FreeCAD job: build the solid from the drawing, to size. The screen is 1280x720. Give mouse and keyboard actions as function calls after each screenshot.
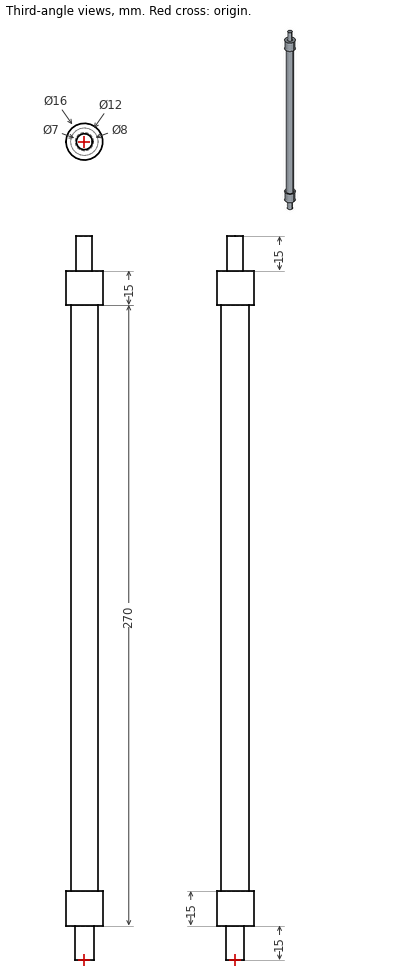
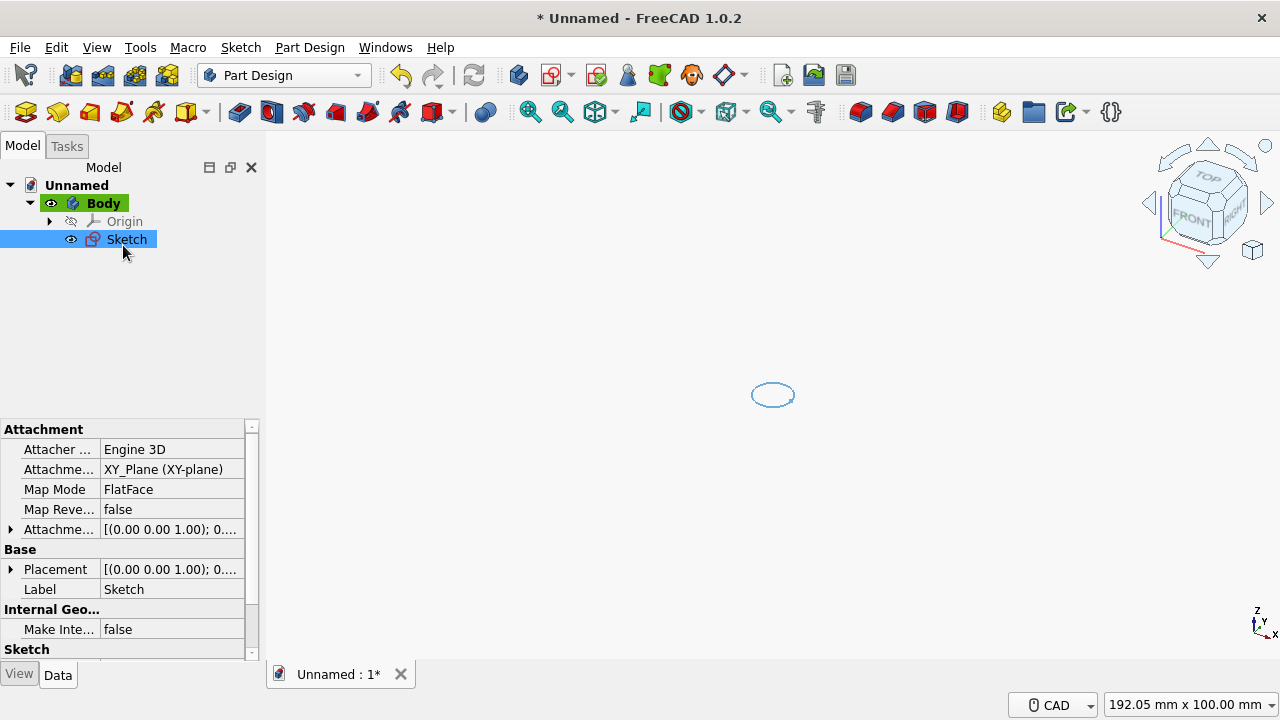
click(26, 112)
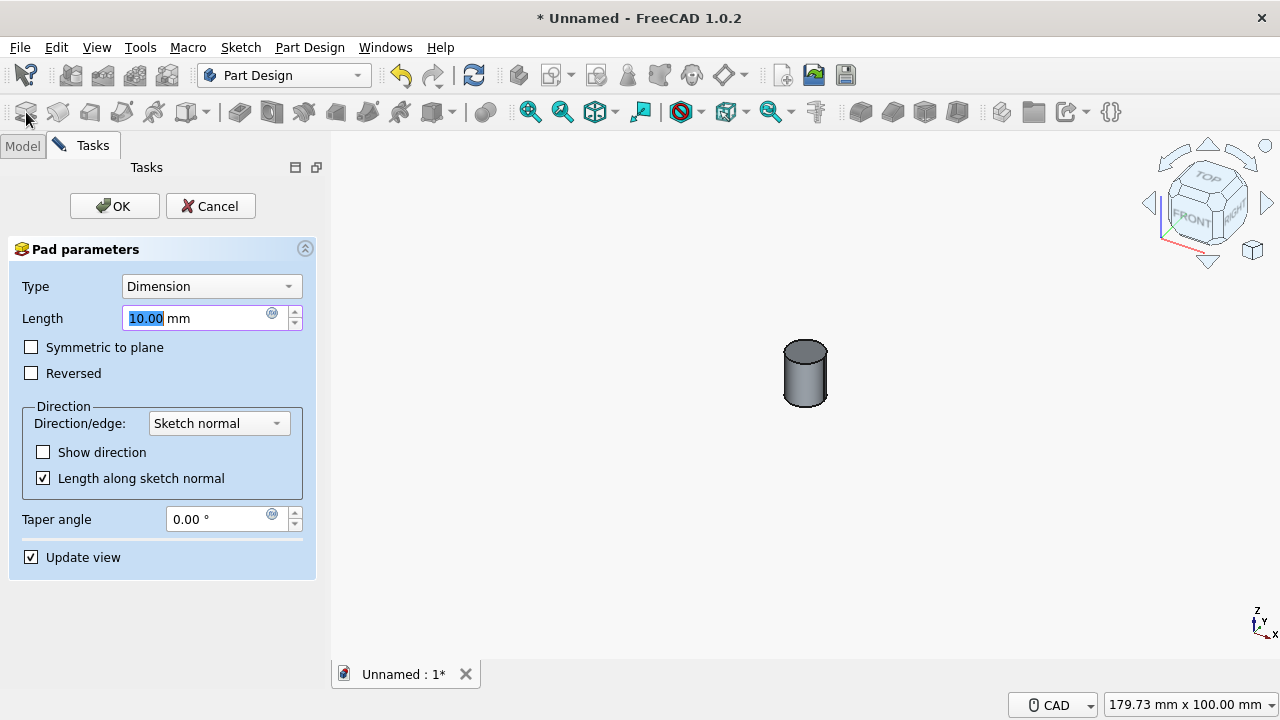
text(15)
key(Tab)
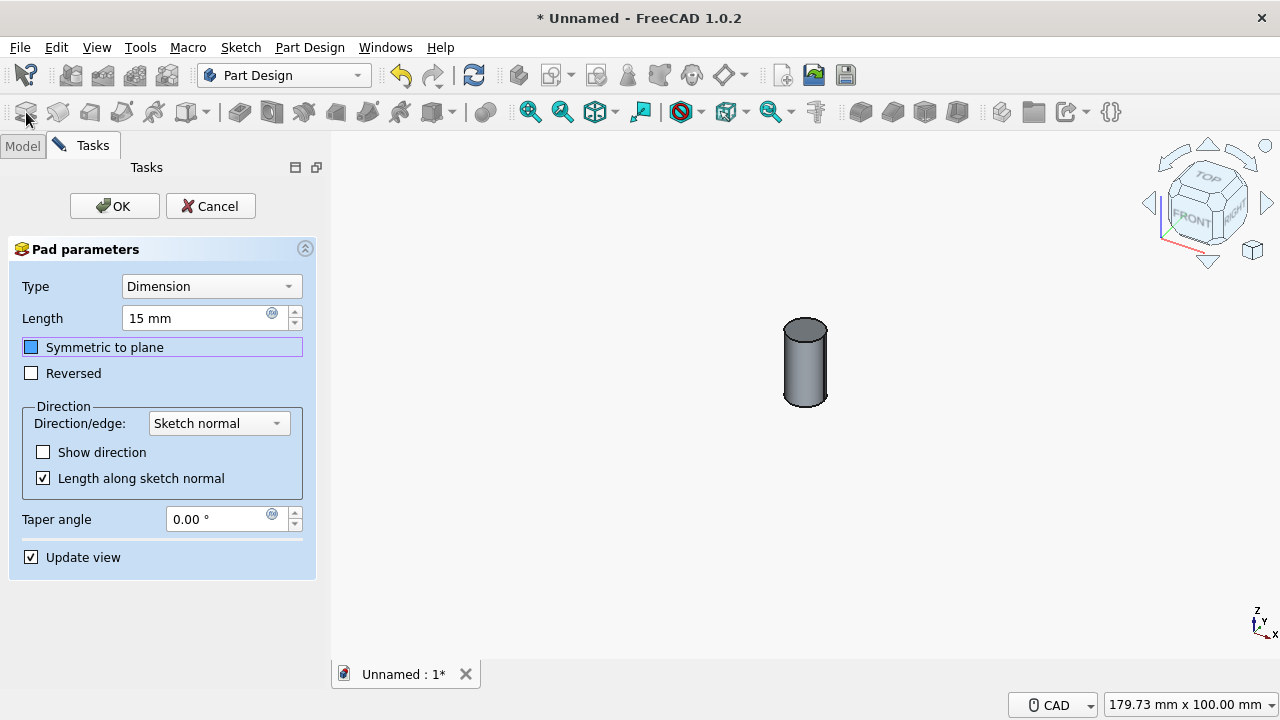
click(115, 206)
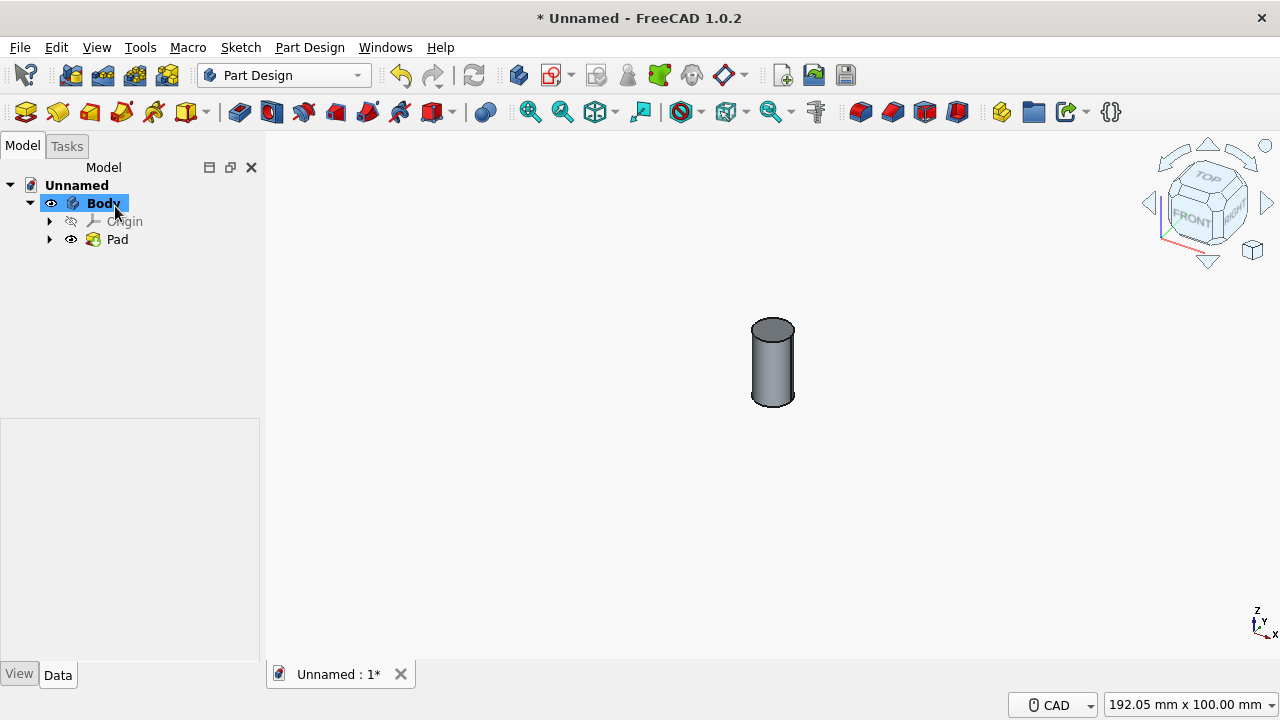
click(532, 112)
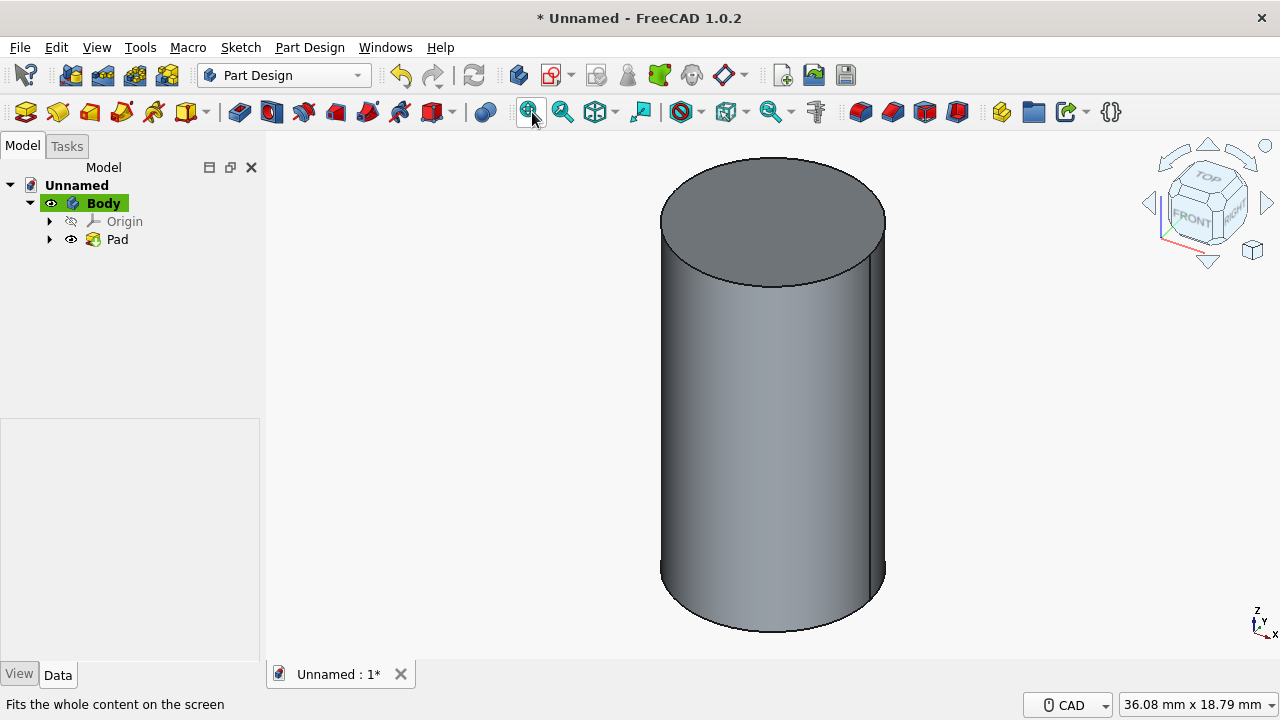
click(773, 221)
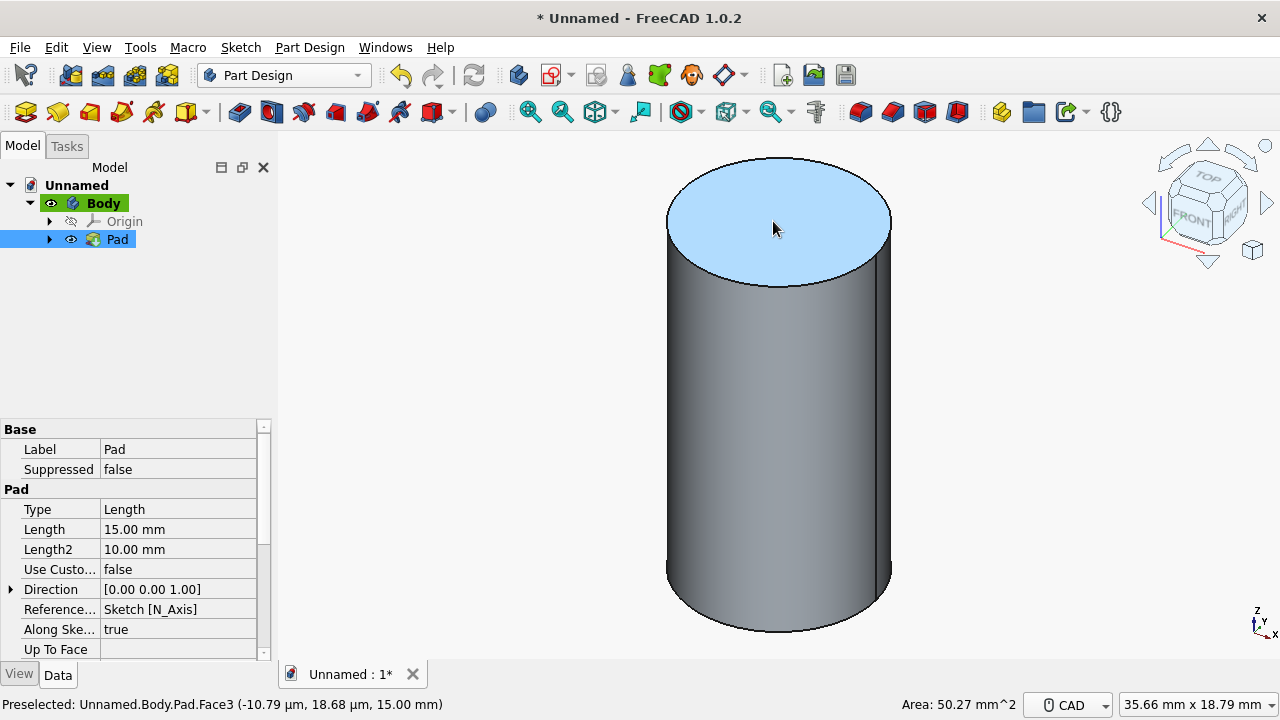
click(552, 76)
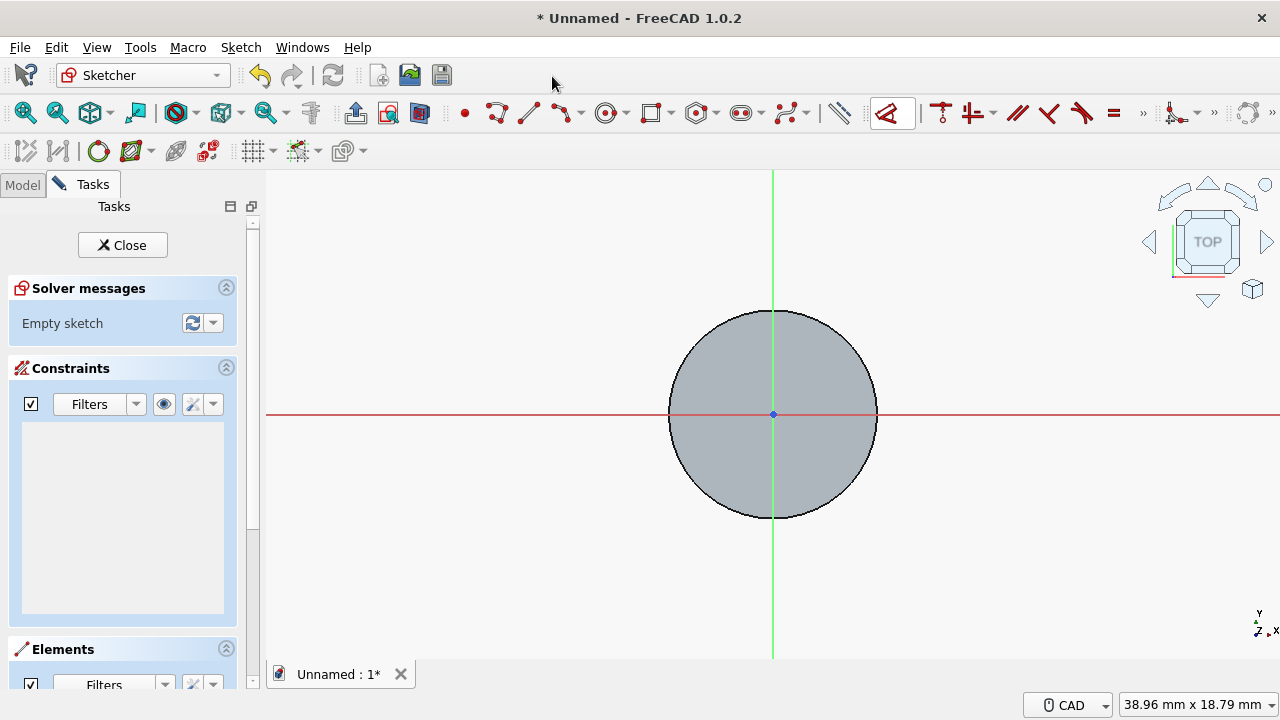
click(606, 114)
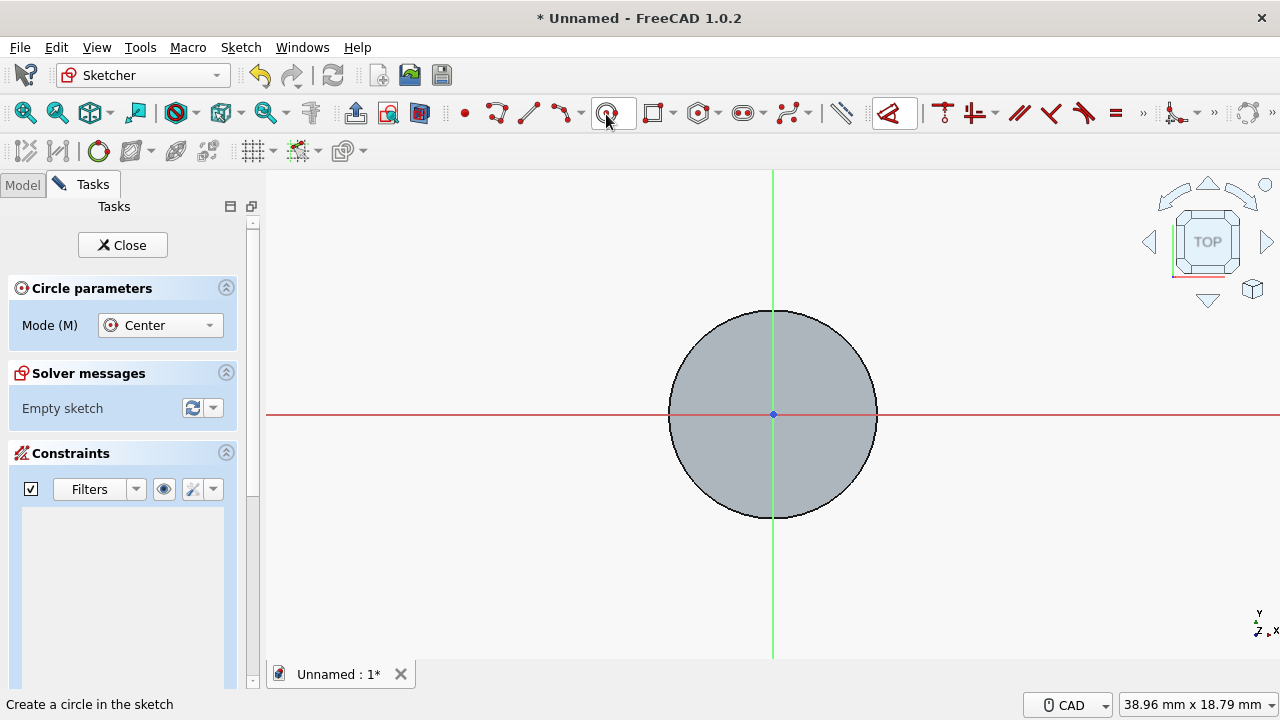
click(773, 414)
click(883, 304)
key(Escape)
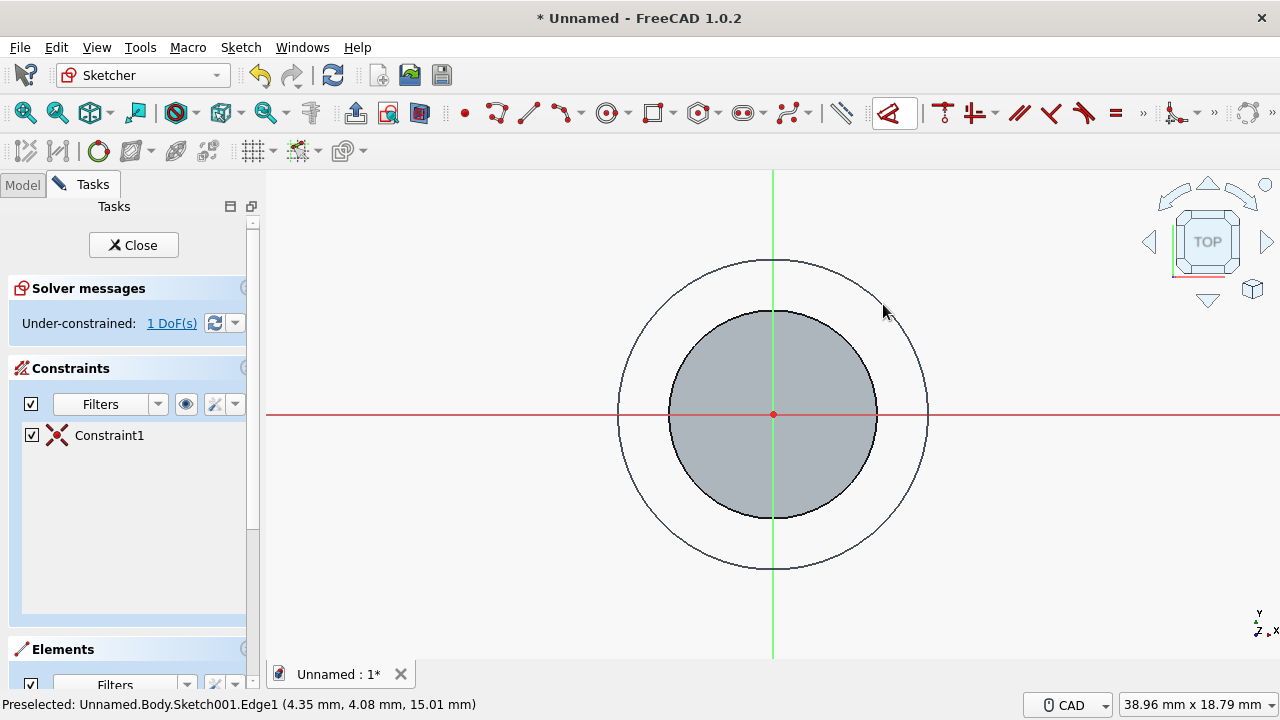
click(882, 304)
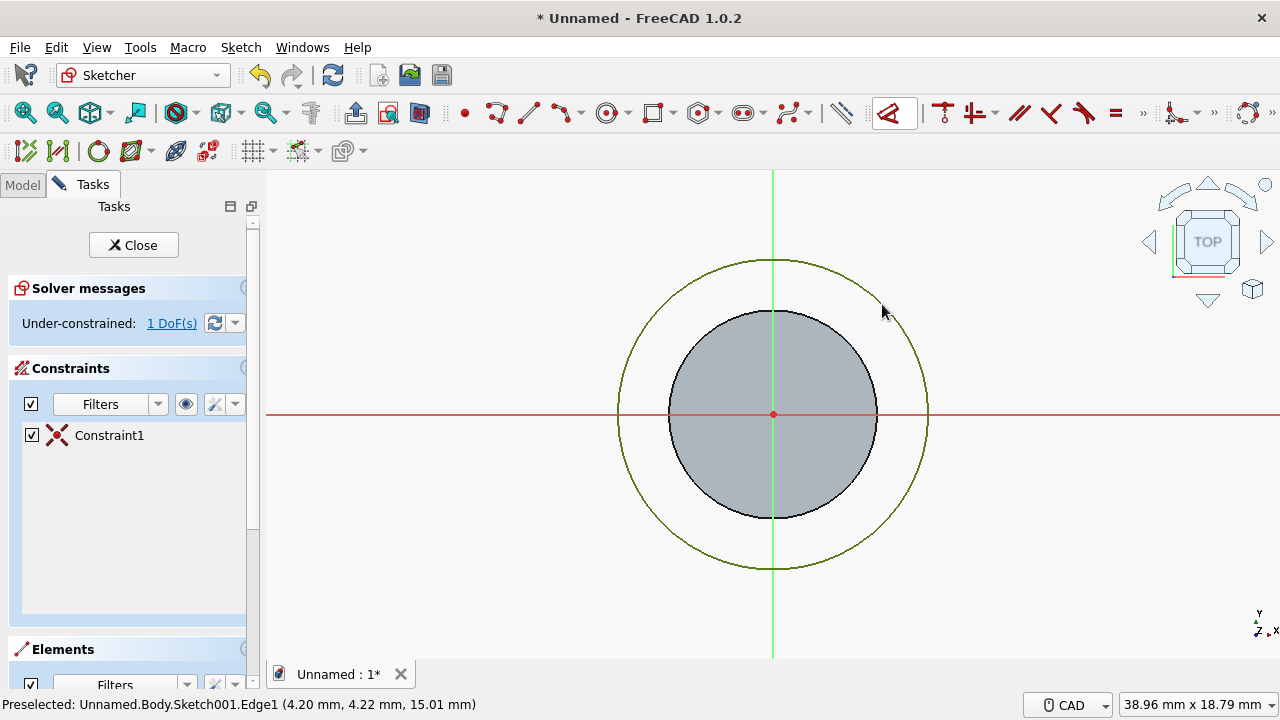
key(k)
key(o)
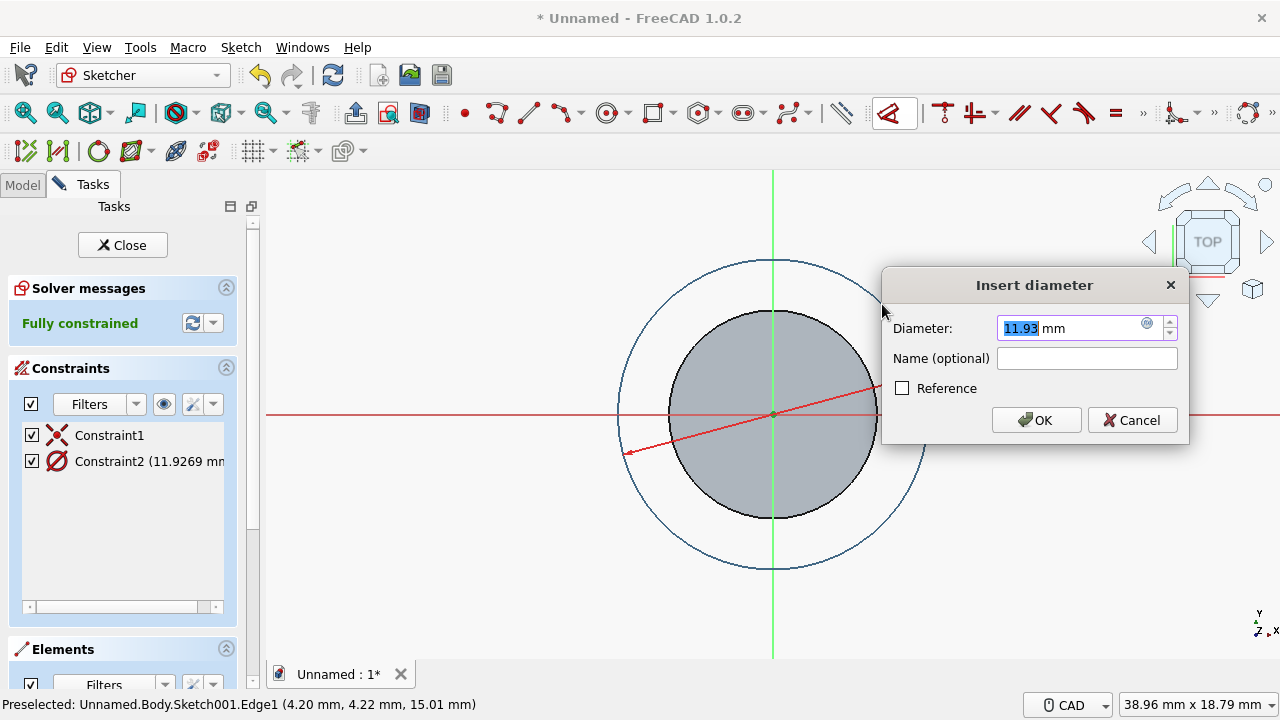
text(12)
key(Return)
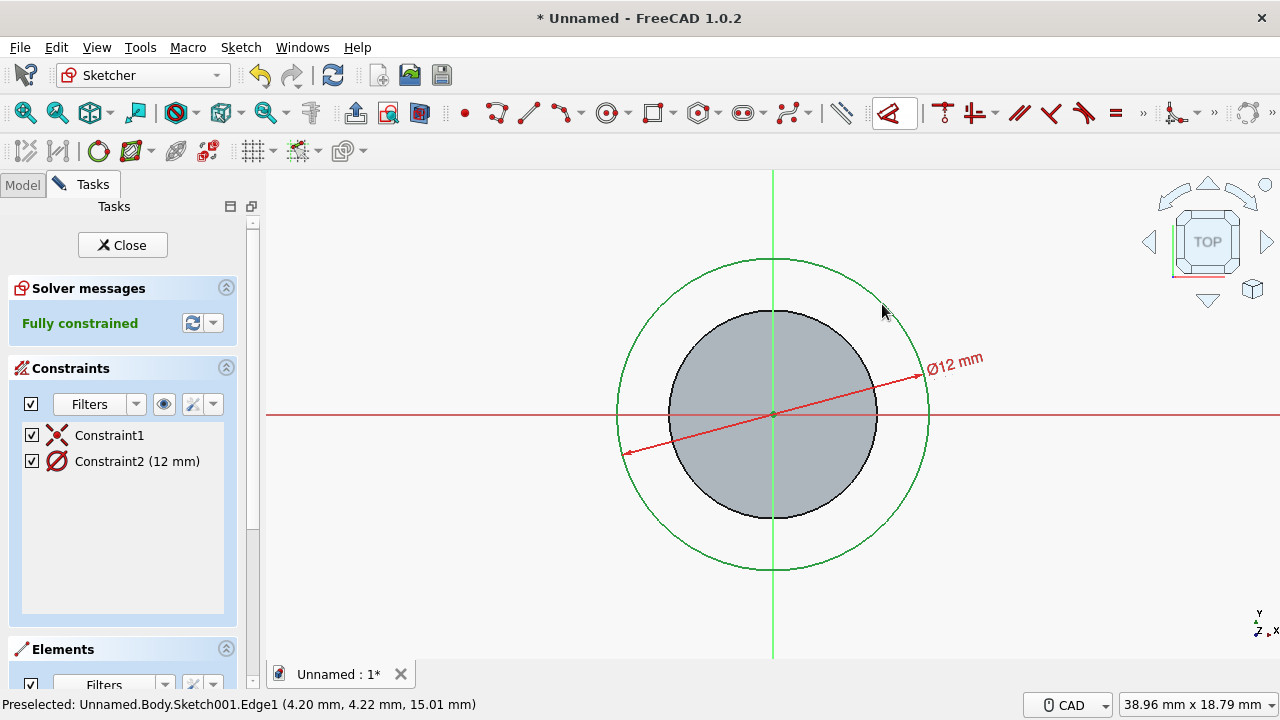
click(123, 245)